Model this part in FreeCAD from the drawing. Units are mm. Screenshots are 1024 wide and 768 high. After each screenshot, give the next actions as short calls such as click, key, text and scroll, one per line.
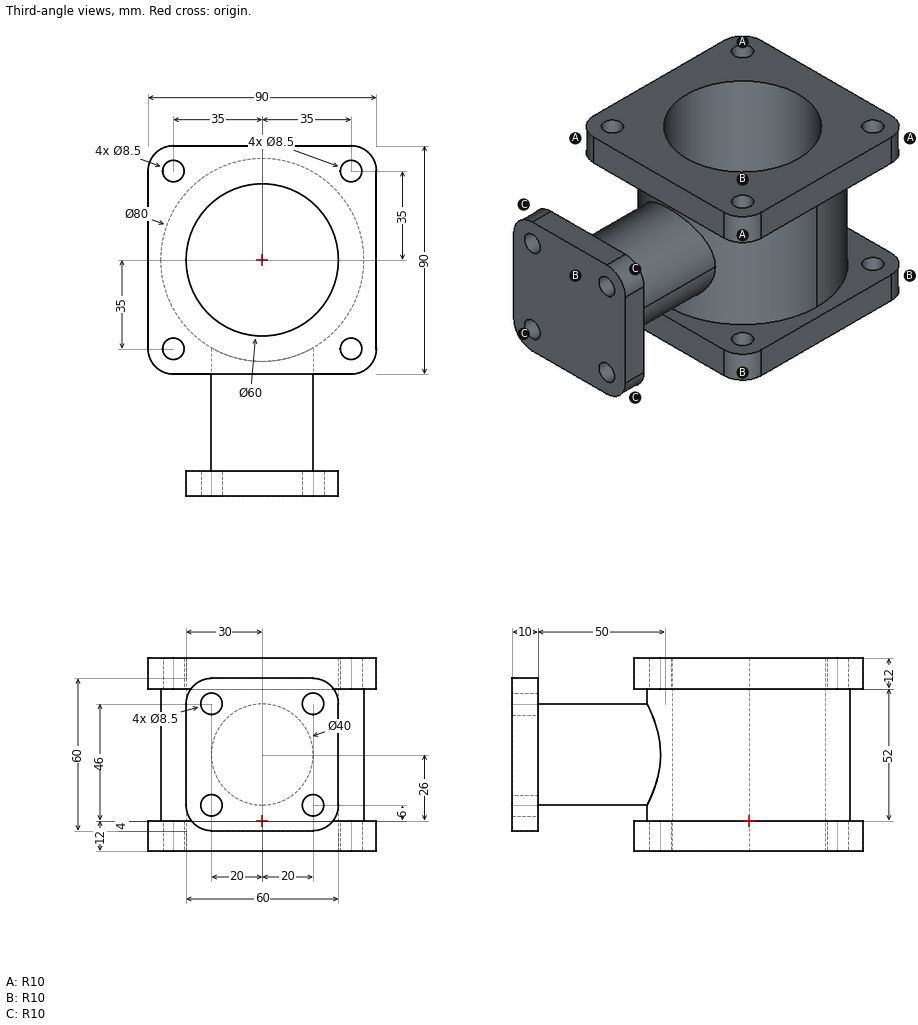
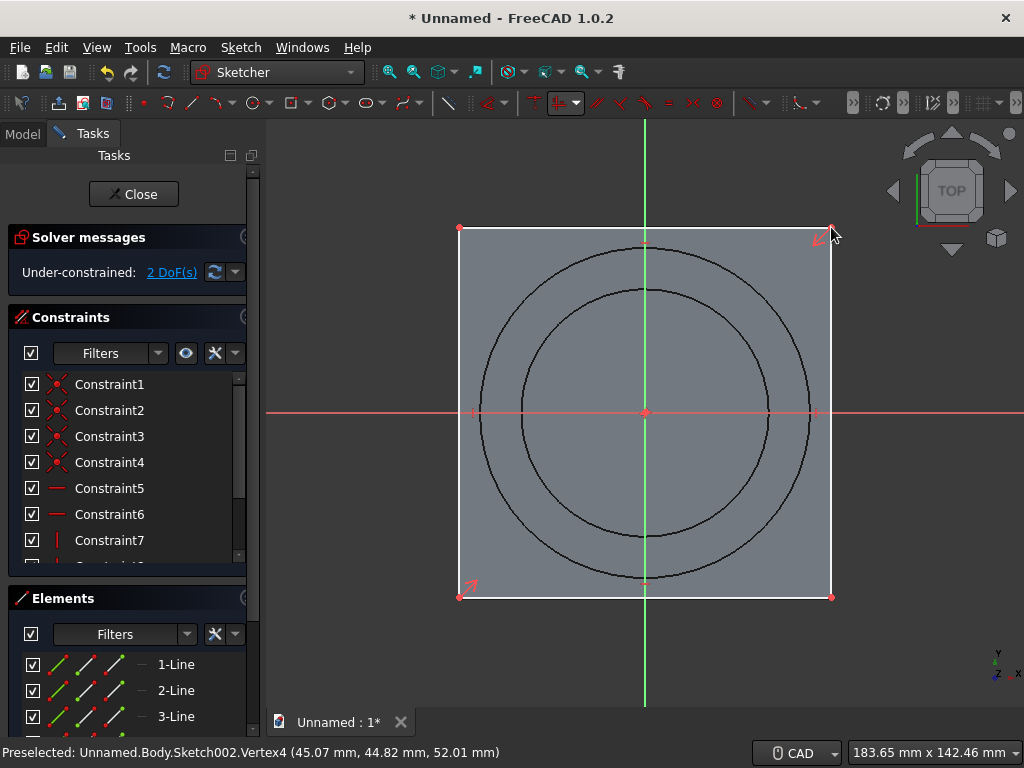
click(488, 104)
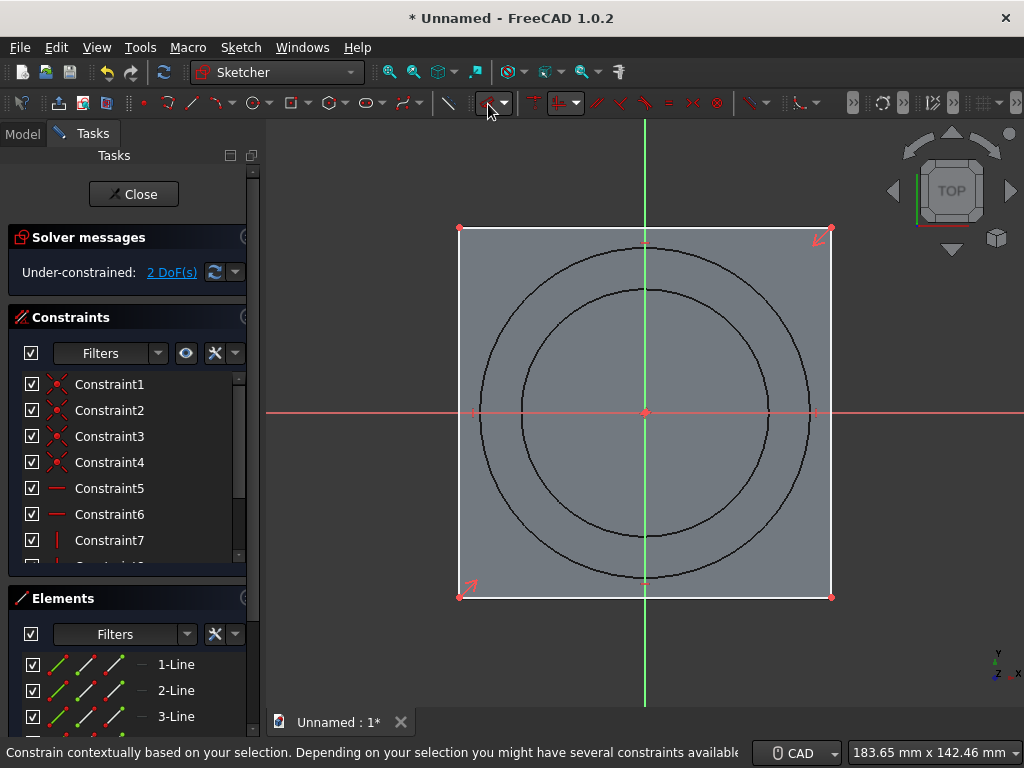
click(571, 598)
click(559, 632)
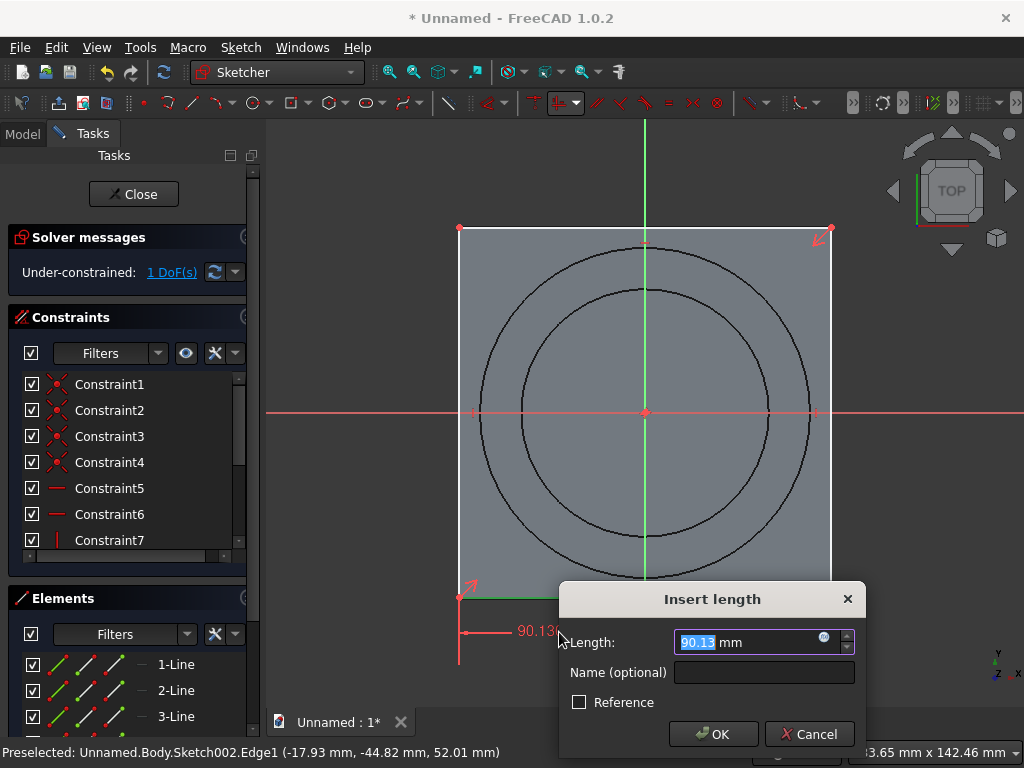
text(90)
key(Return)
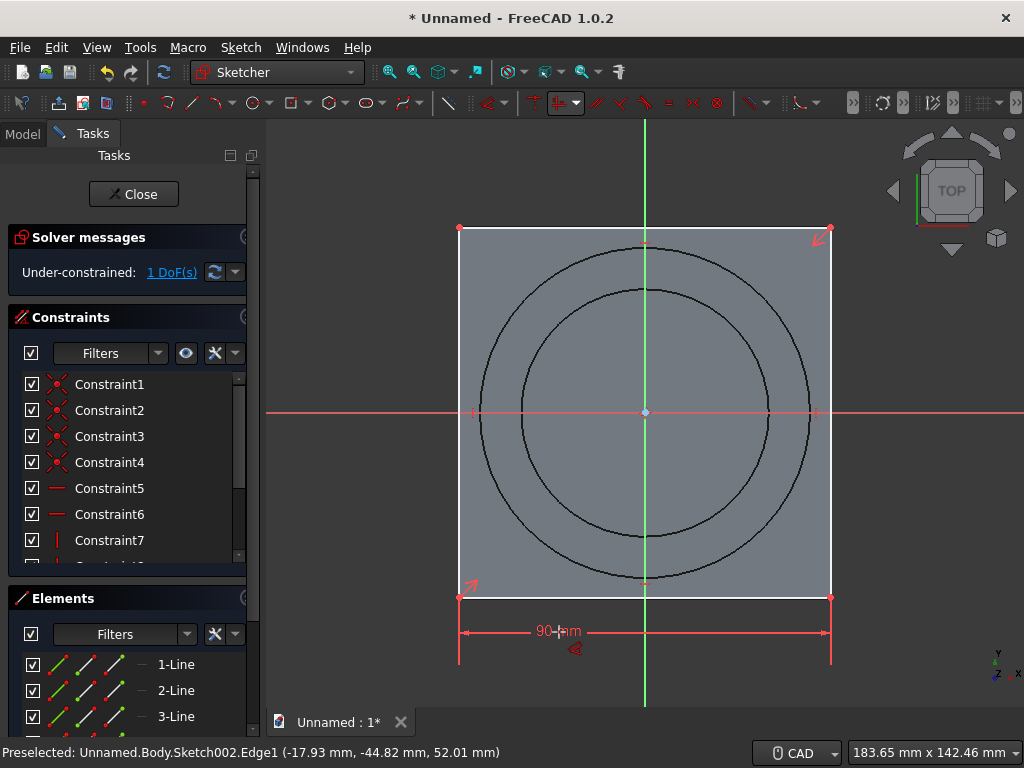
click(831, 487)
click(797, 328)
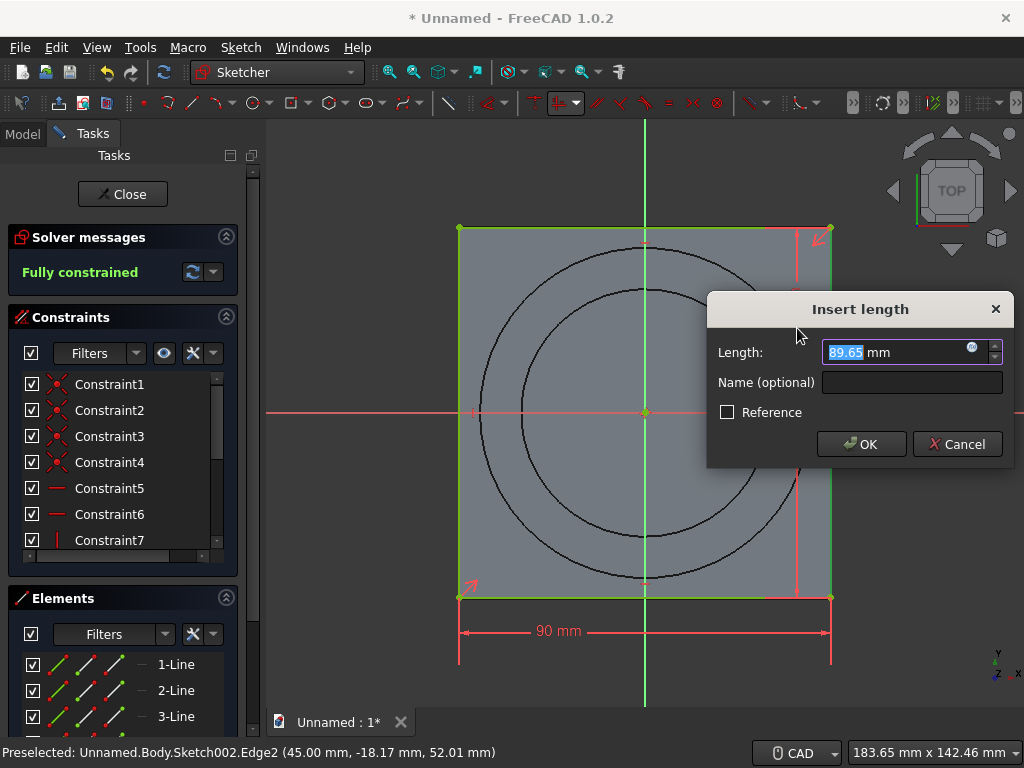
text(90)
key(Return)
key(Escape)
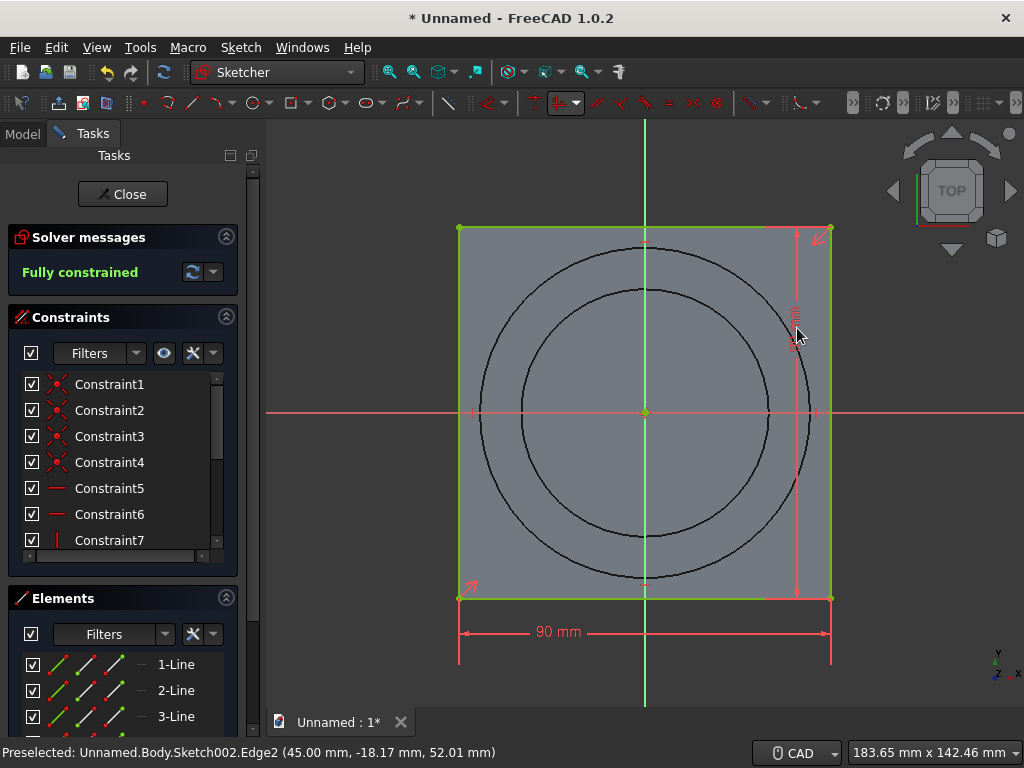
click(123, 194)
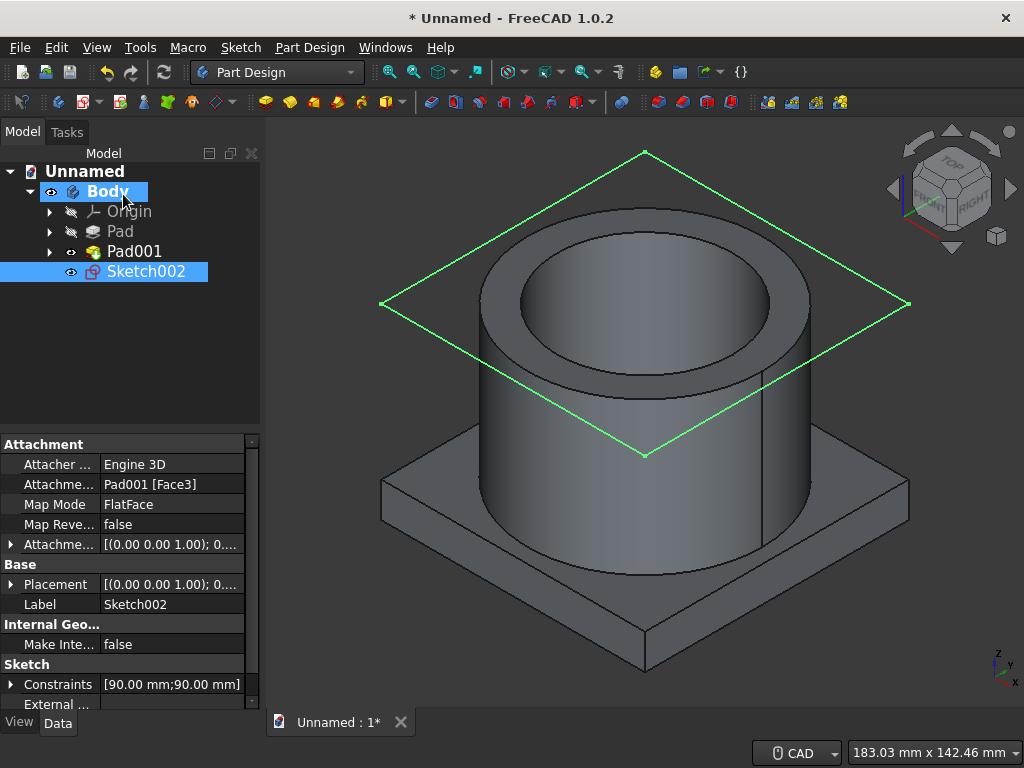
click(266, 102)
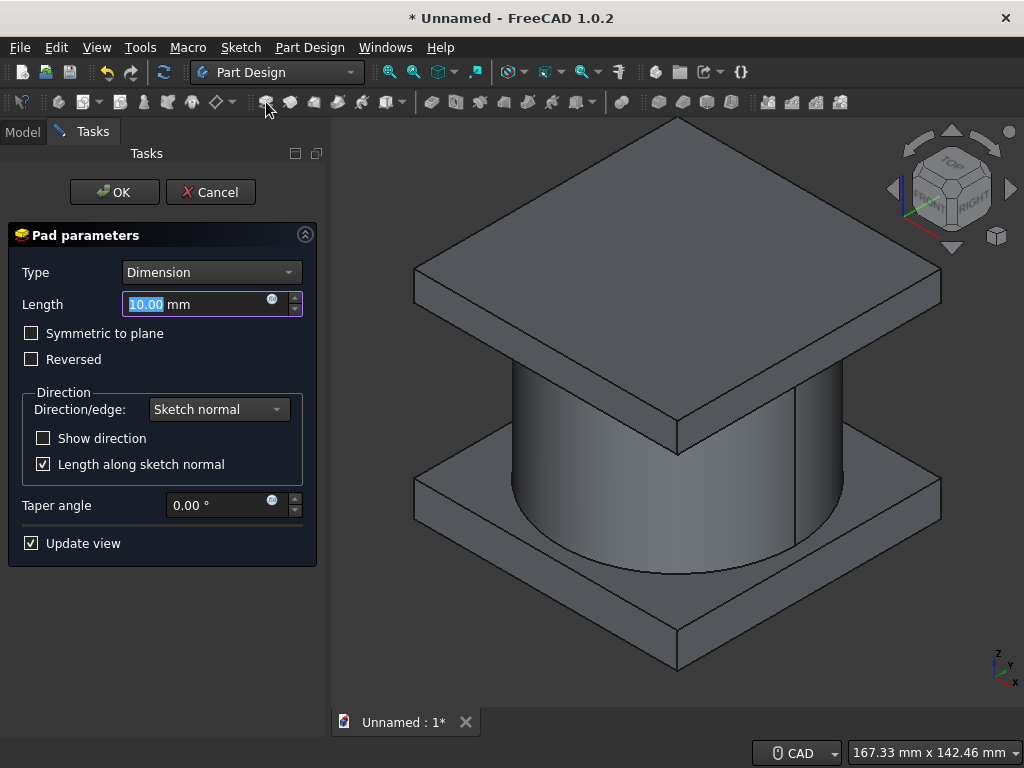
text(12)
key(Tab)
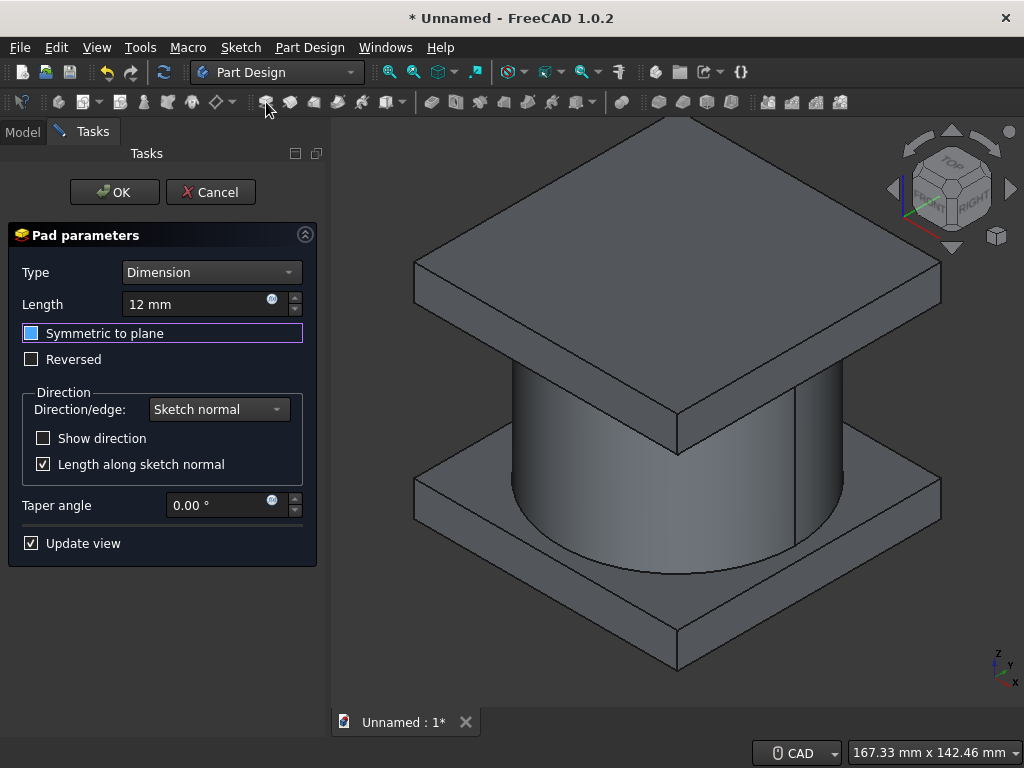
click(115, 192)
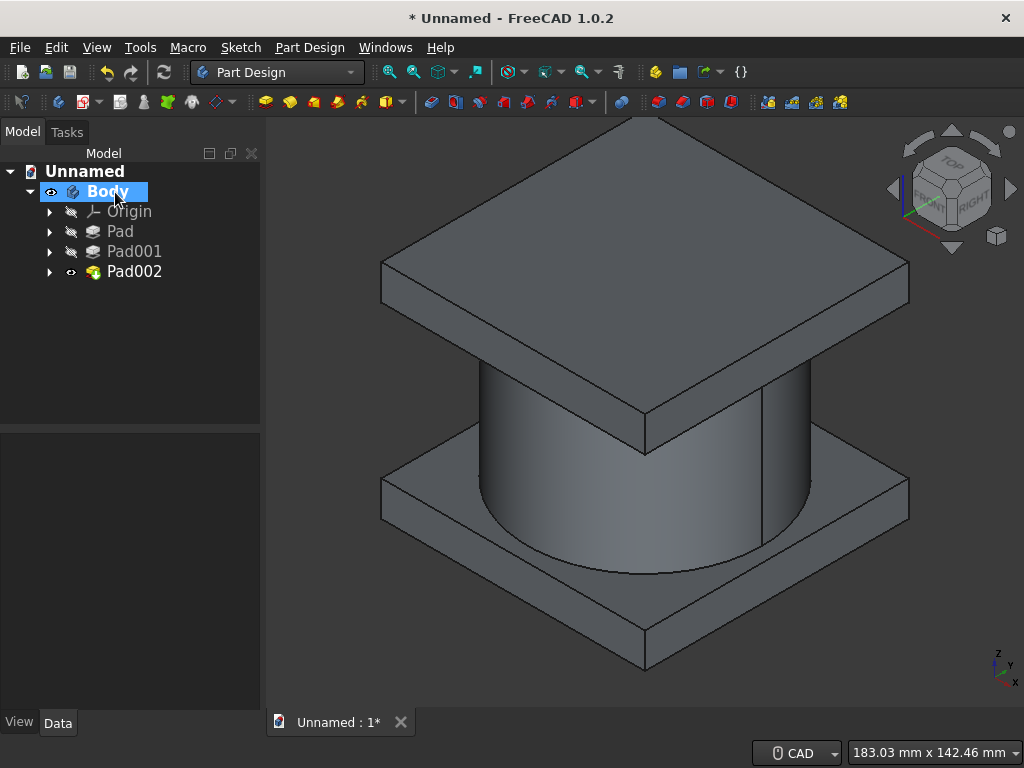
click(390, 72)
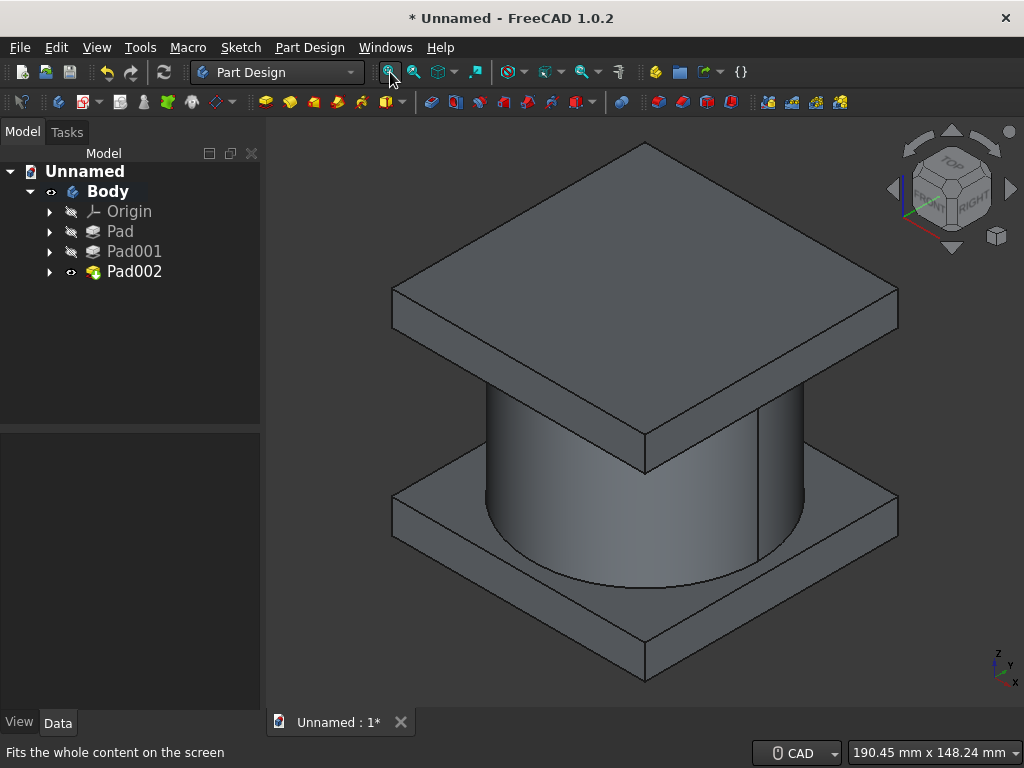
click(645, 288)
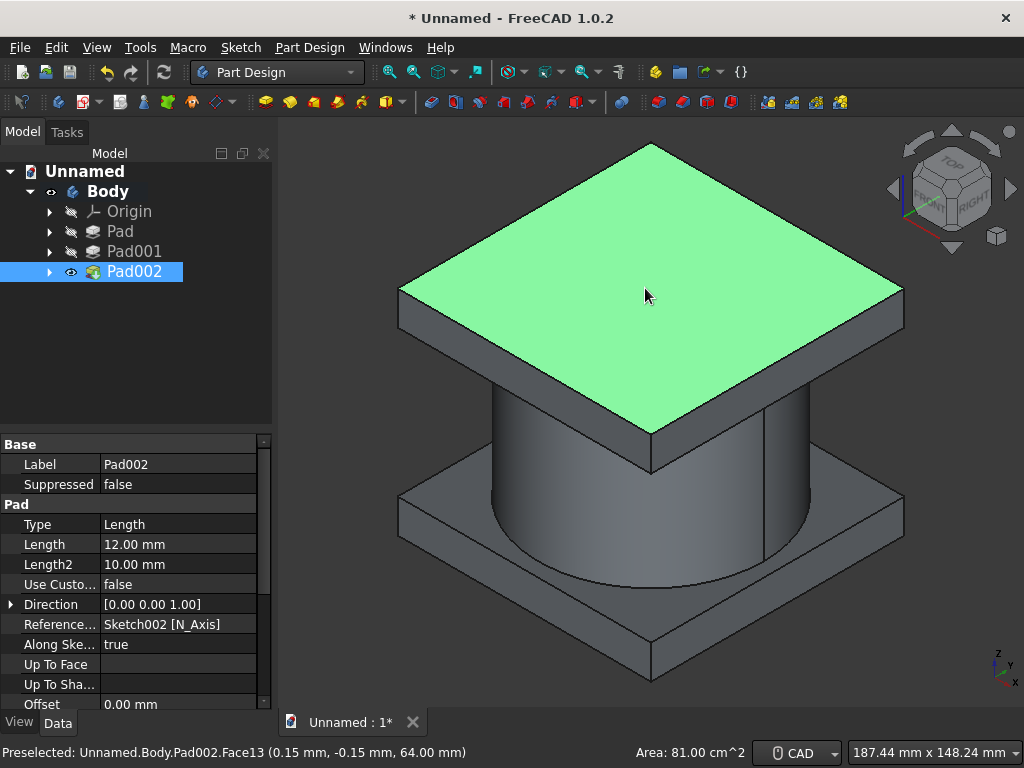
click(84, 102)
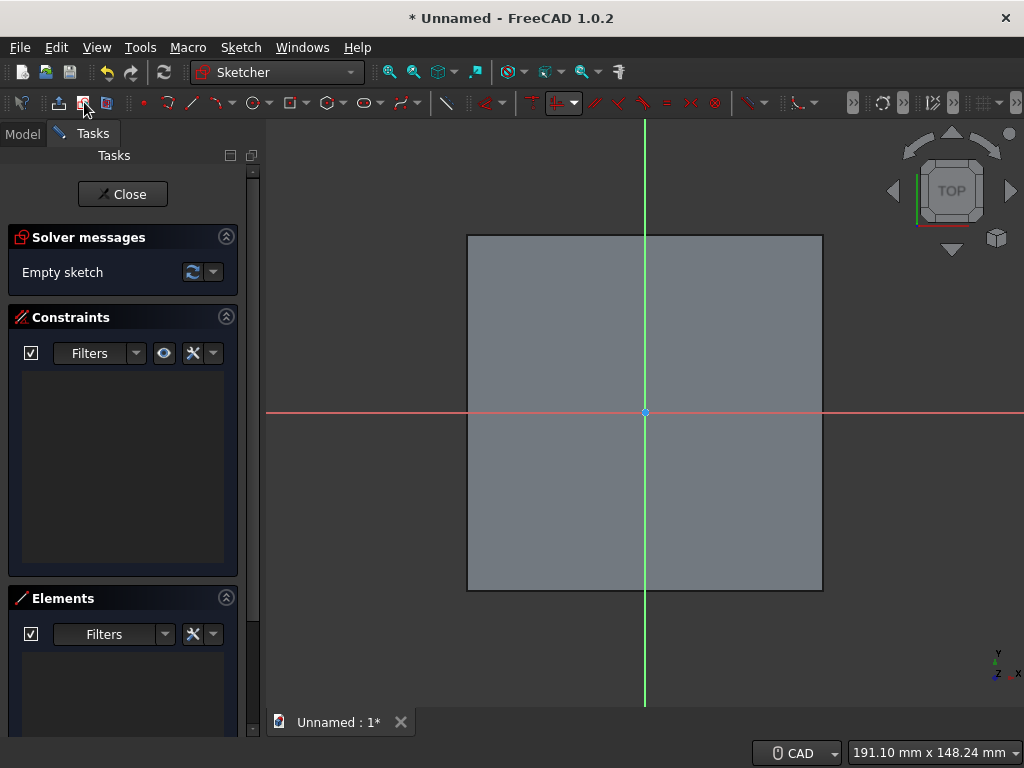
scroll(784, 413, up, 2)